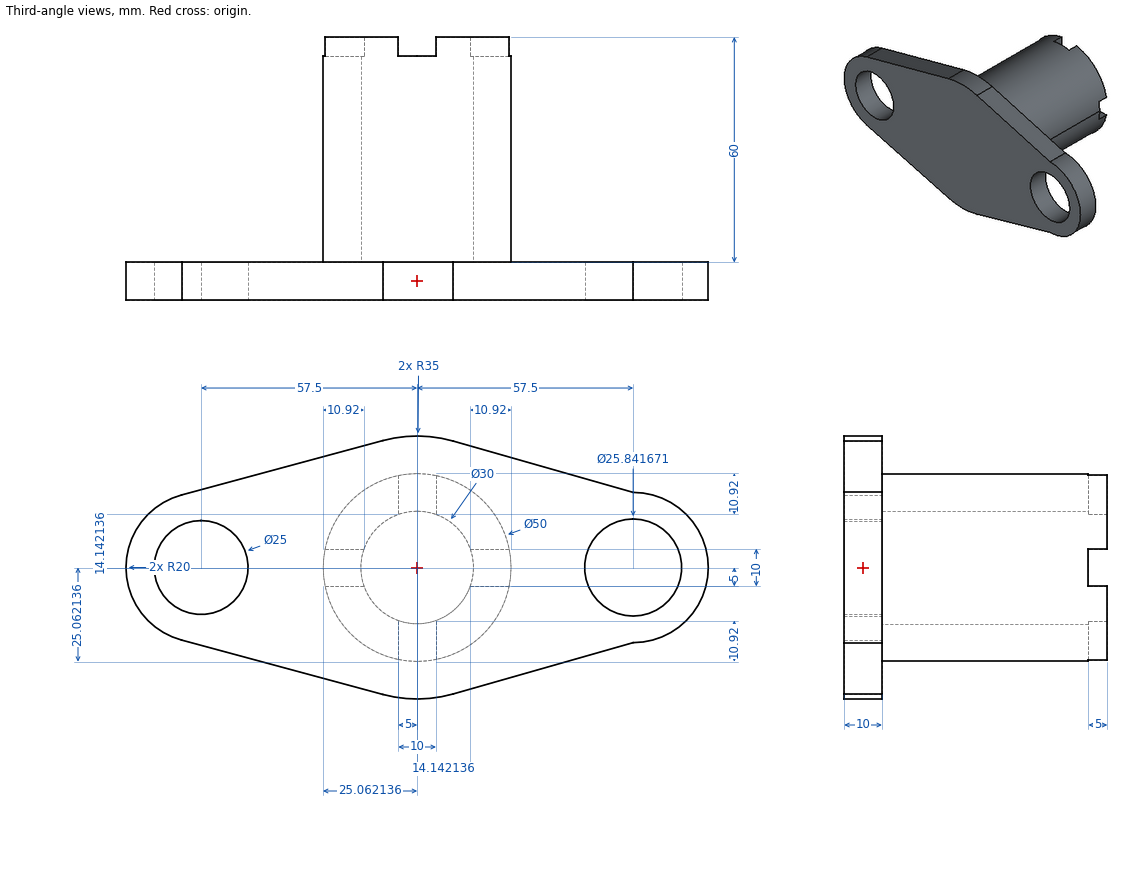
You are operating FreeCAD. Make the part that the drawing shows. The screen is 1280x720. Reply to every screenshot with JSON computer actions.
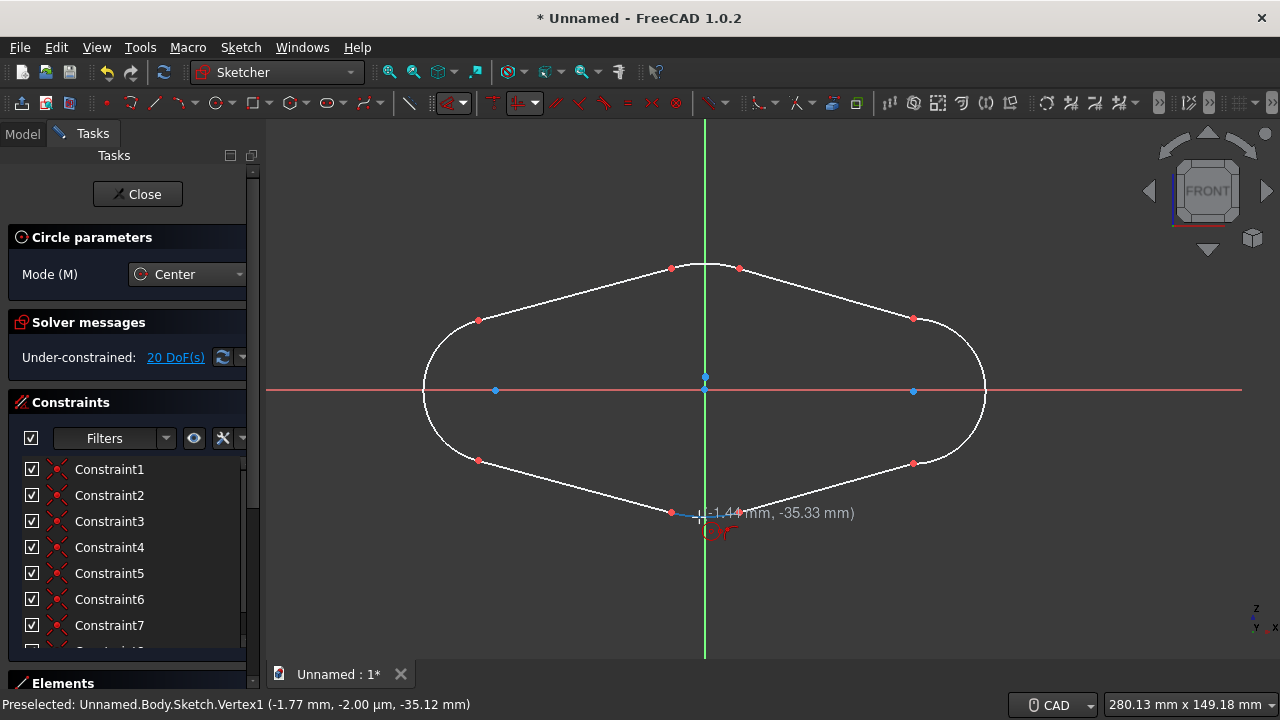
{"action": "left_click", "coordinate": [913, 390]}
{"action": "mouse_move", "coordinate": [946, 357]}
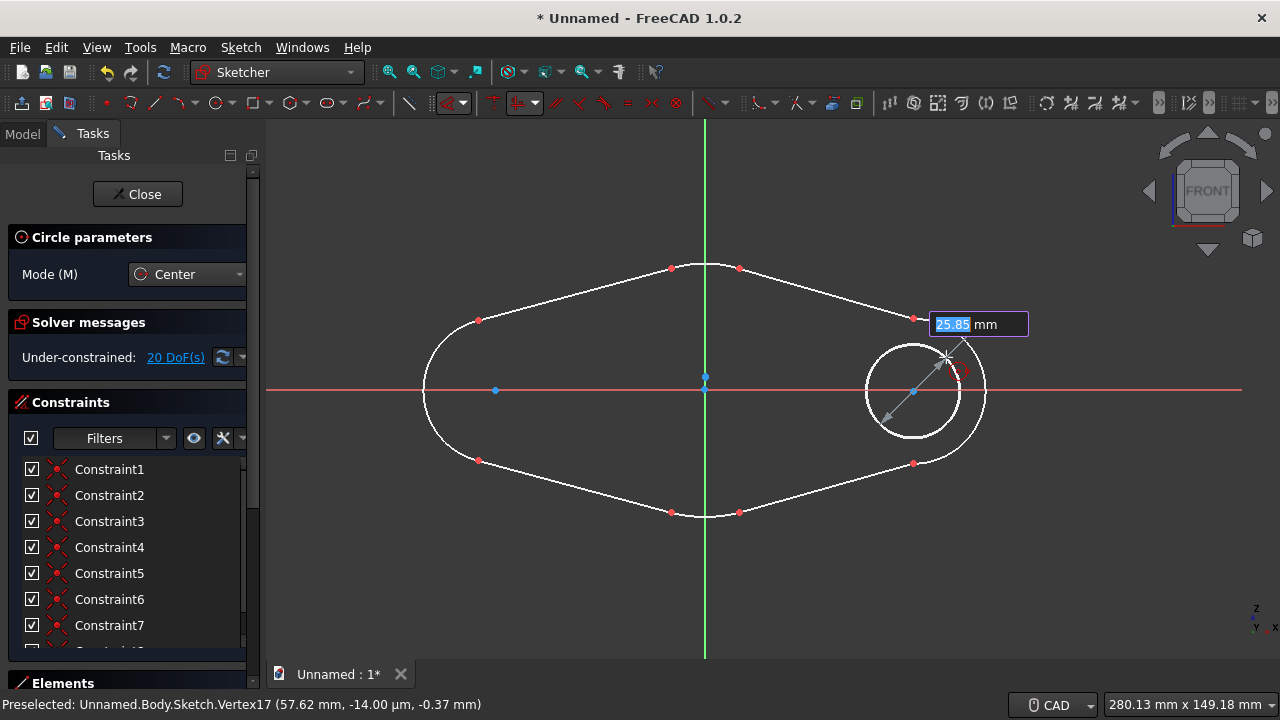
{"action": "type", "text": "25.841671"}
{"action": "key", "text": "Return"}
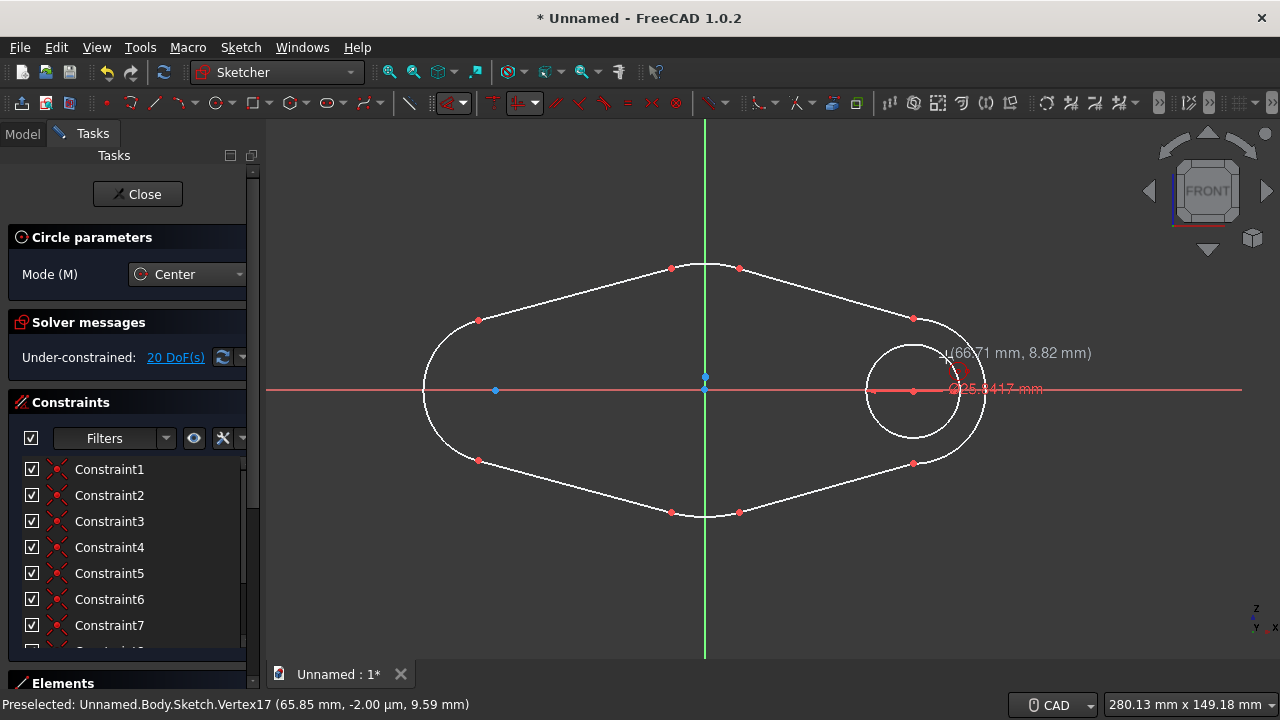
{"action": "left_click", "coordinate": [496, 390]}
{"action": "mouse_move", "coordinate": [528, 358]}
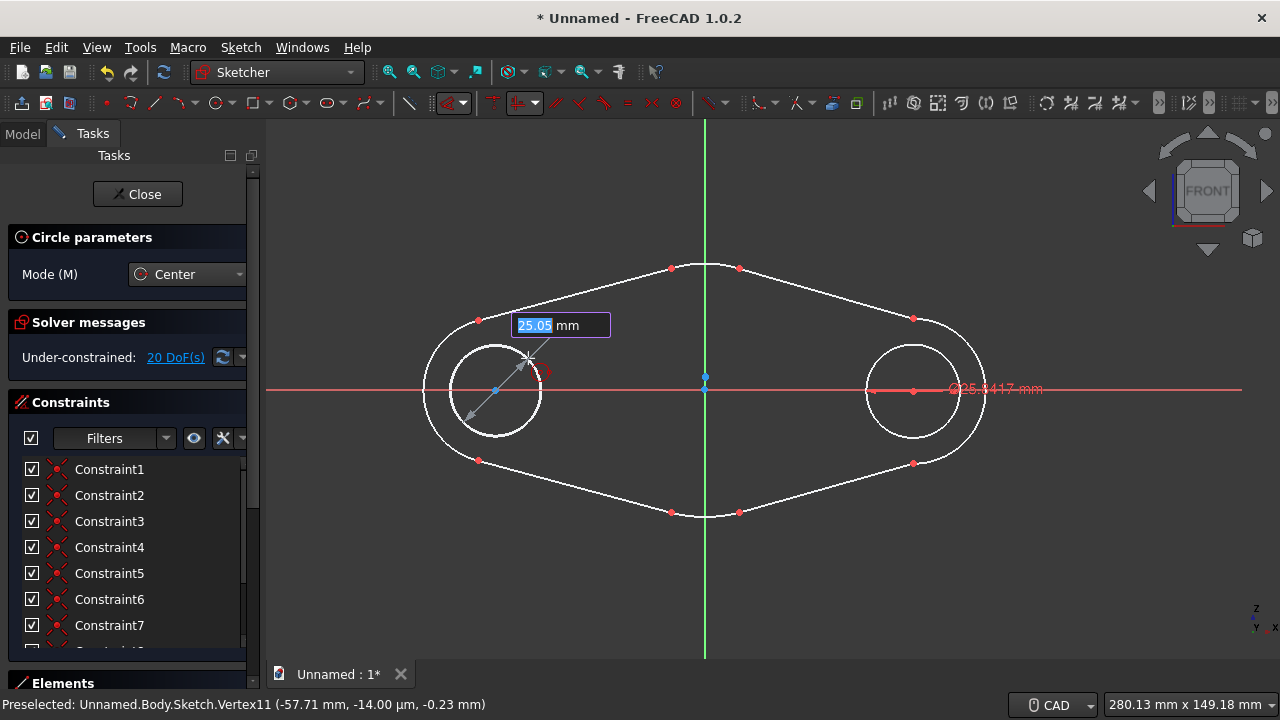
{"action": "type", "text": "25"}
{"action": "key", "text": "Return"}
{"action": "key", "text": "Escape"}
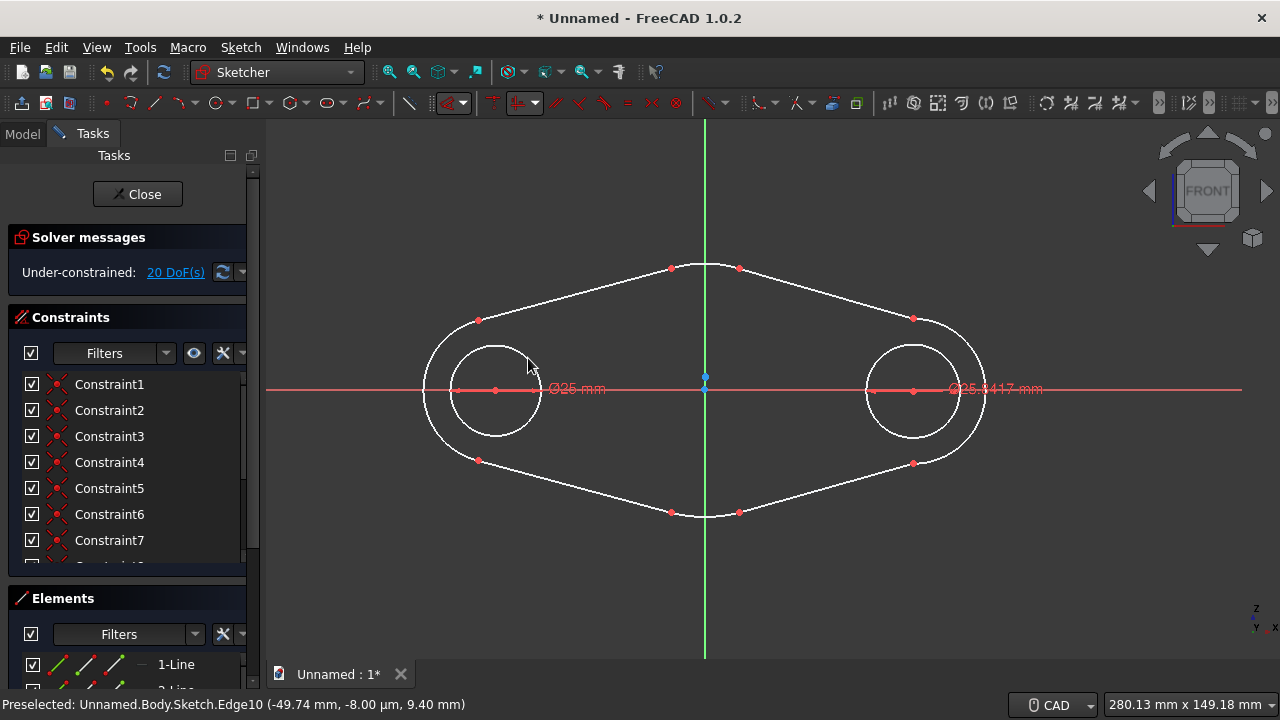
{"action": "left_click", "coordinate": [613, 497]}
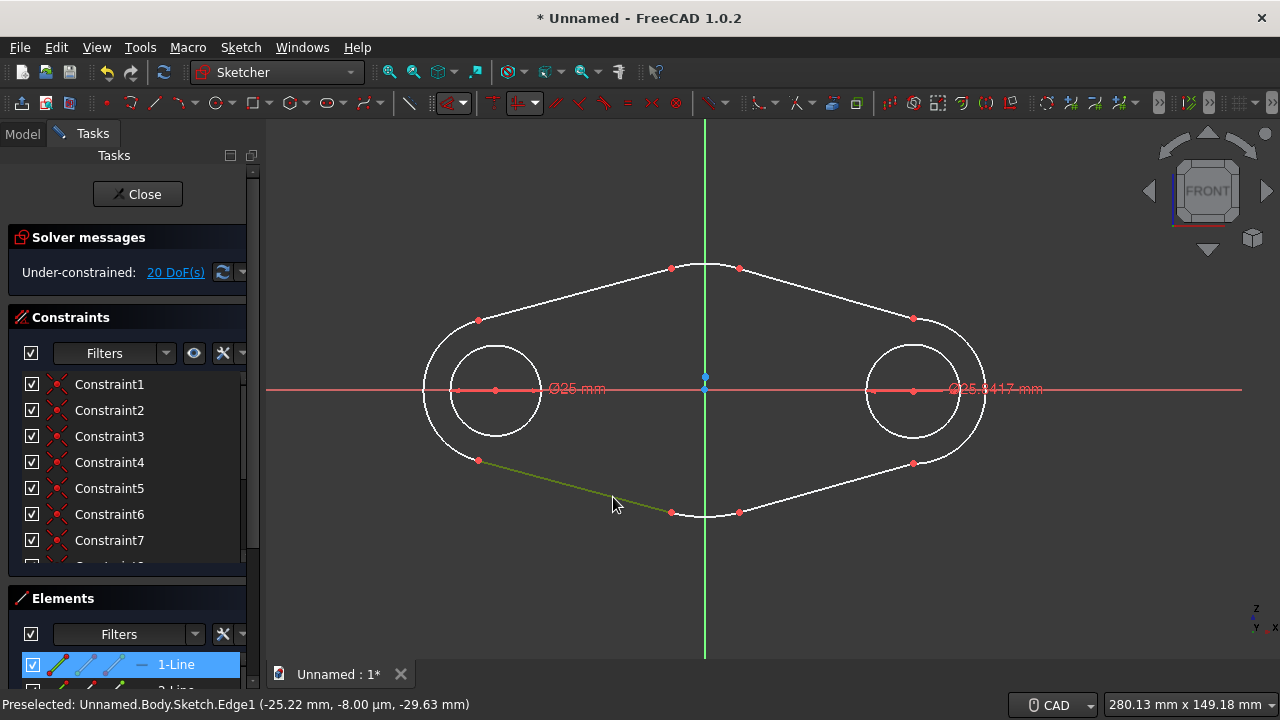
{"action": "left_click", "coordinate": [433, 354]}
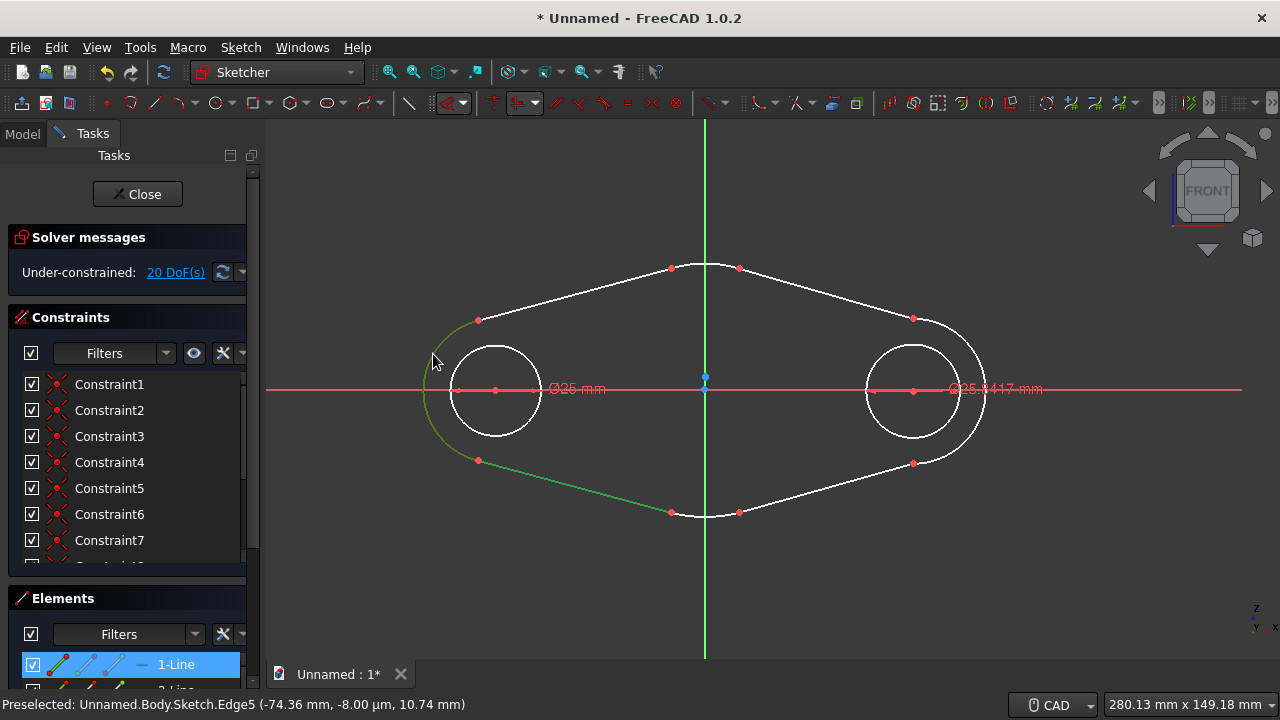
{"action": "key", "text": "t"}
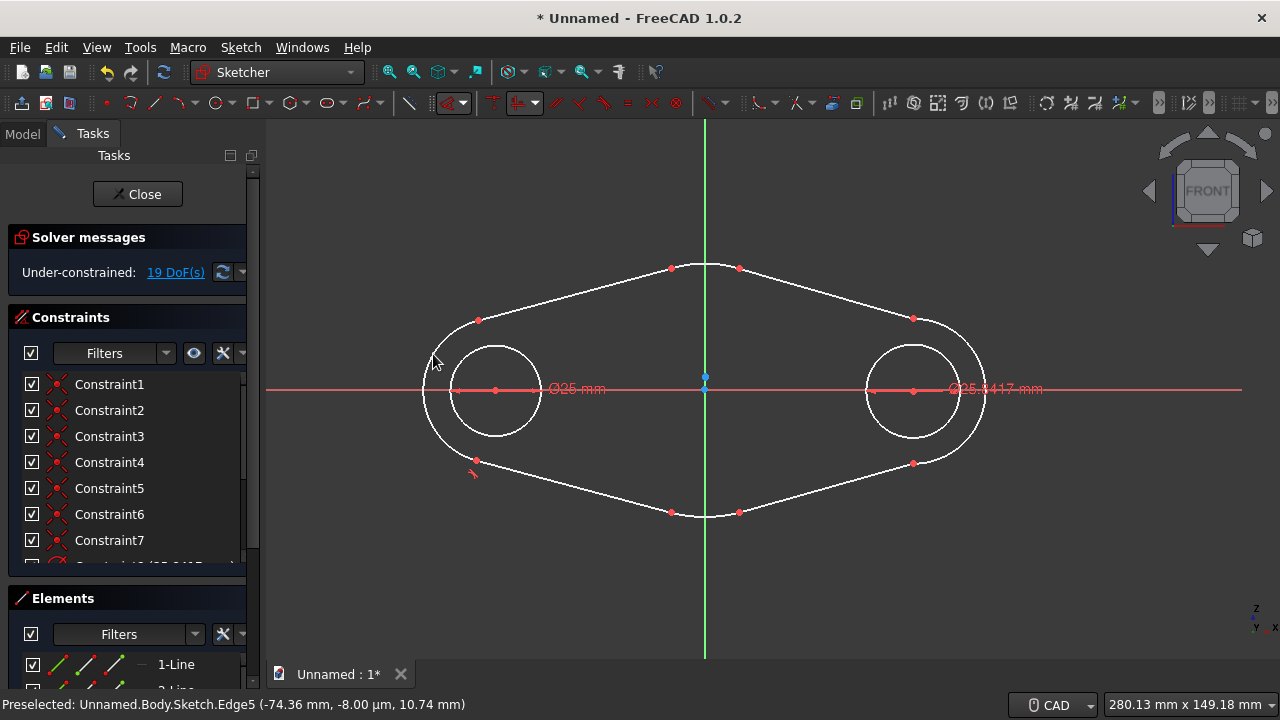
{"action": "left_click", "coordinate": [613, 497]}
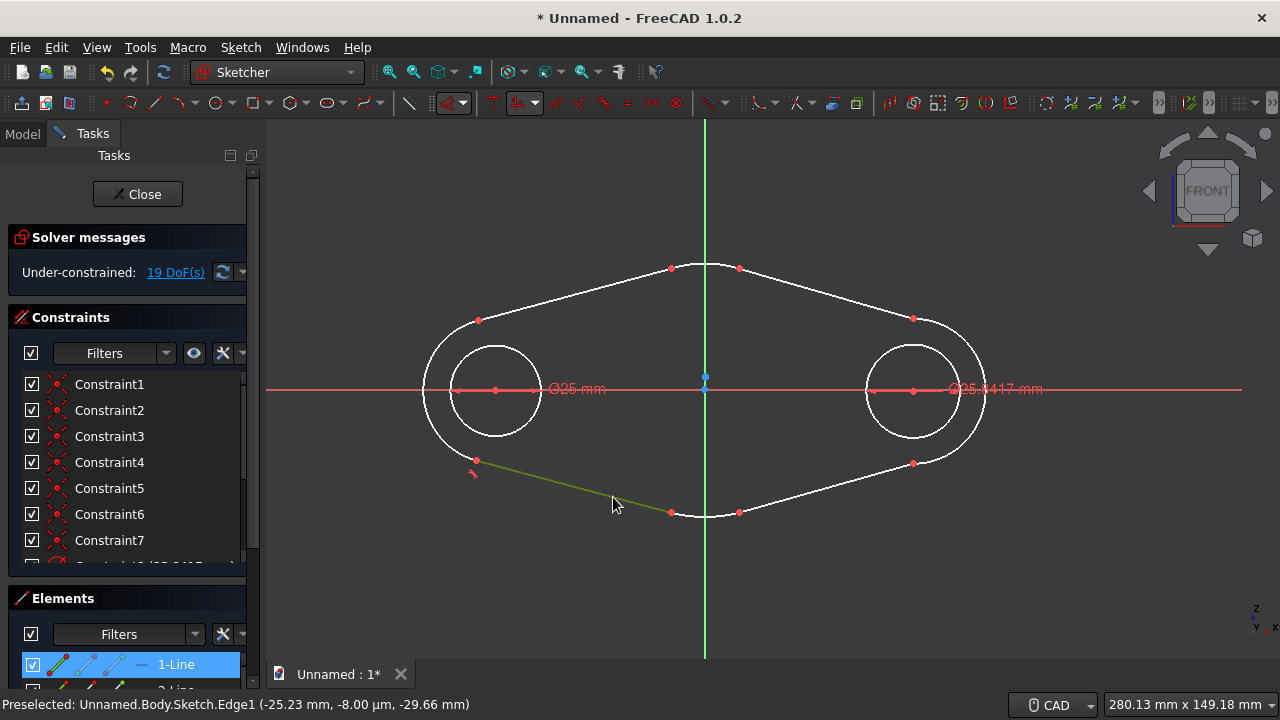
{"action": "left_click", "coordinate": [691, 516]}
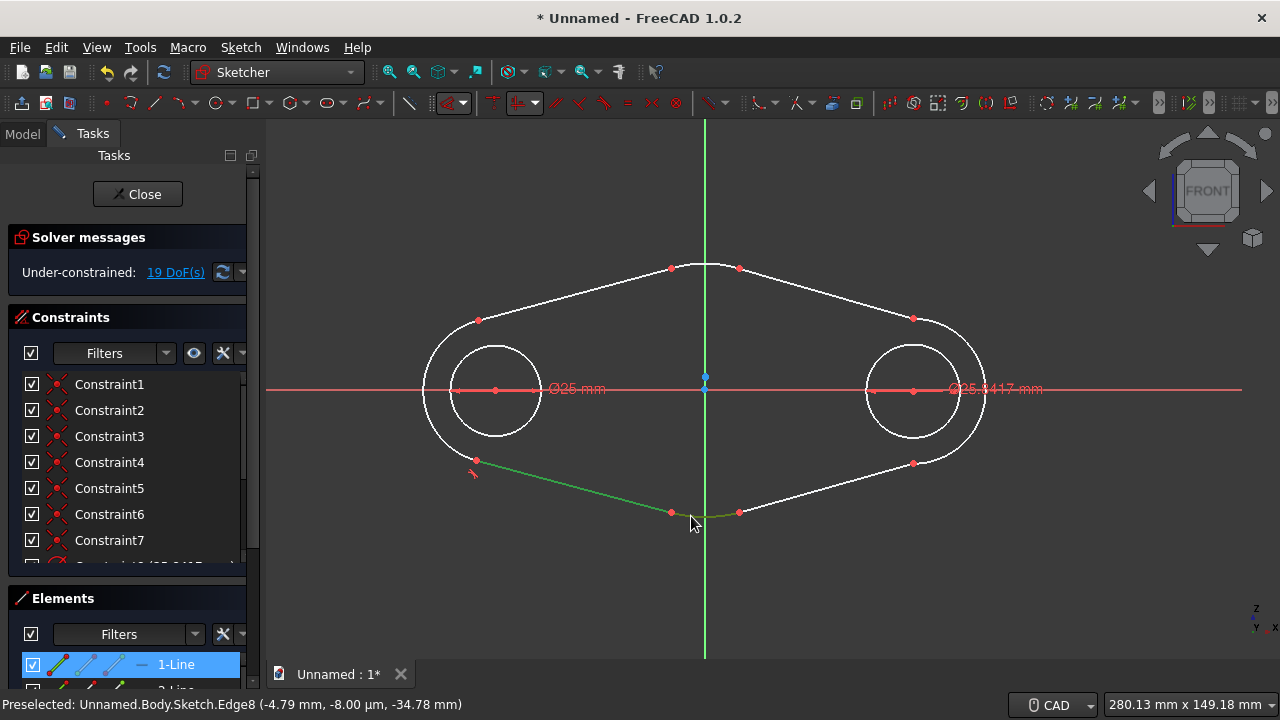
{"action": "left_click", "coordinate": [604, 104]}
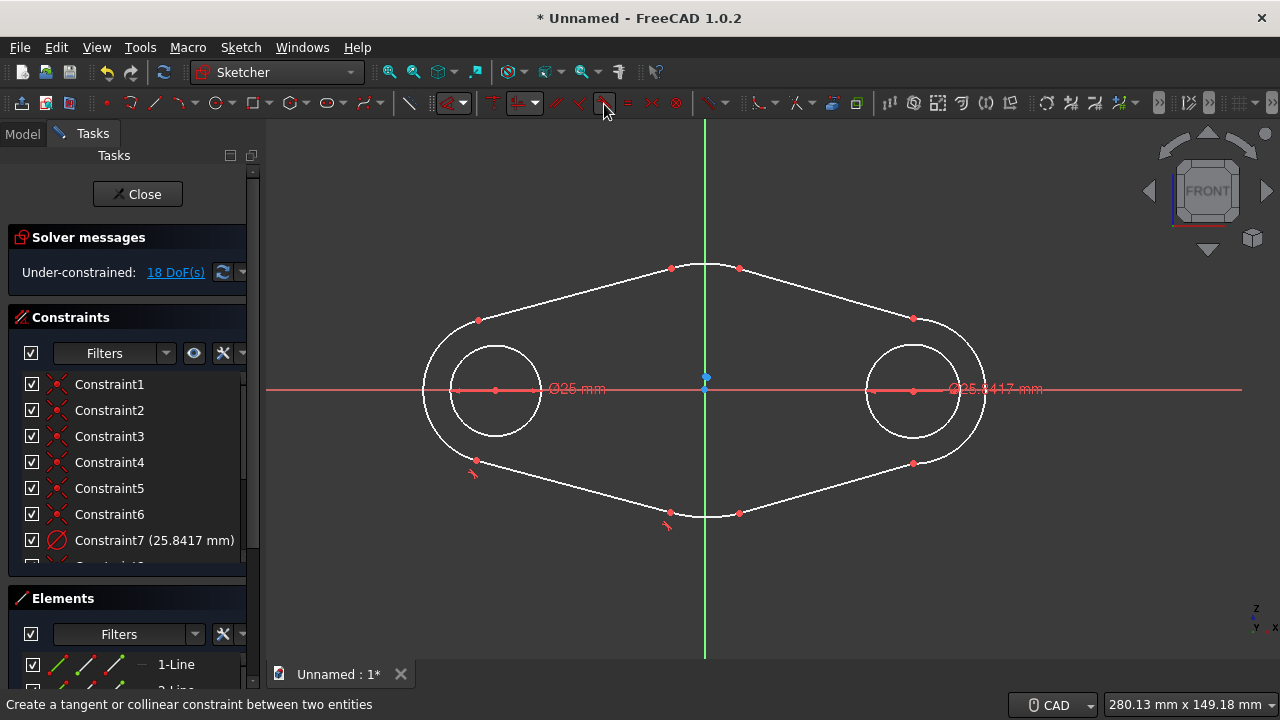
{"action": "left_click", "coordinate": [536, 305]}